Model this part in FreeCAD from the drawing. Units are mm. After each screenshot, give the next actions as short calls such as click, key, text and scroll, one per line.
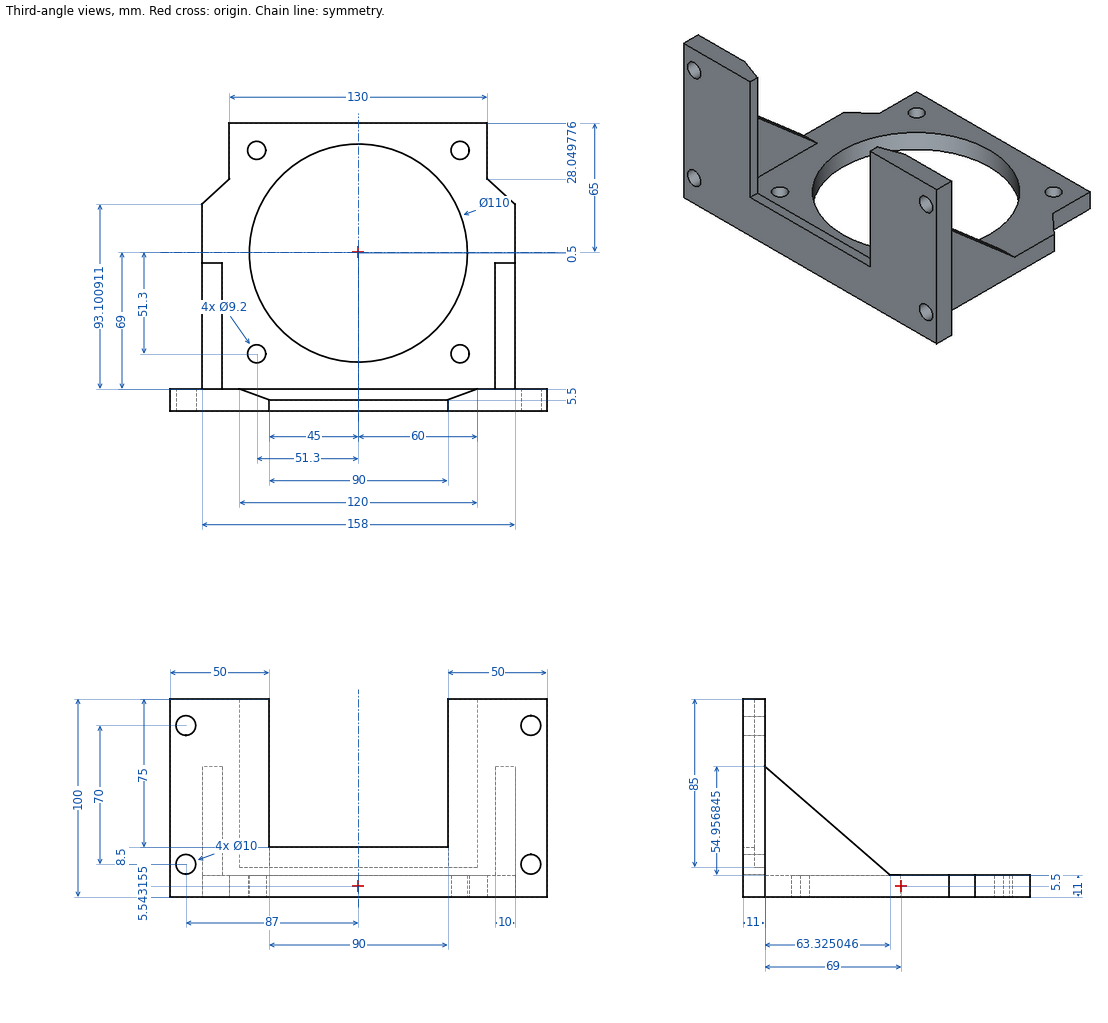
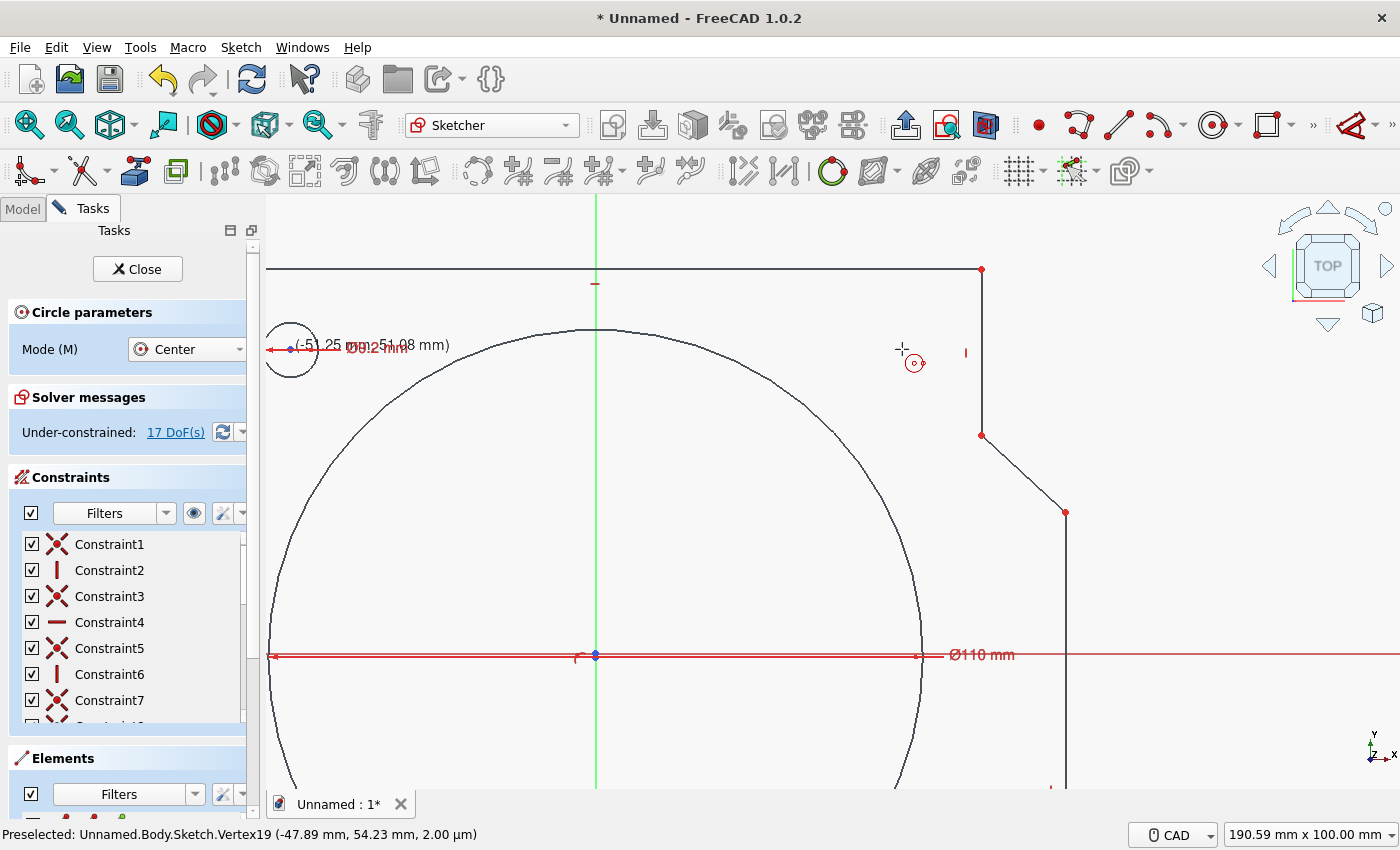
click(901, 349)
move(920, 329)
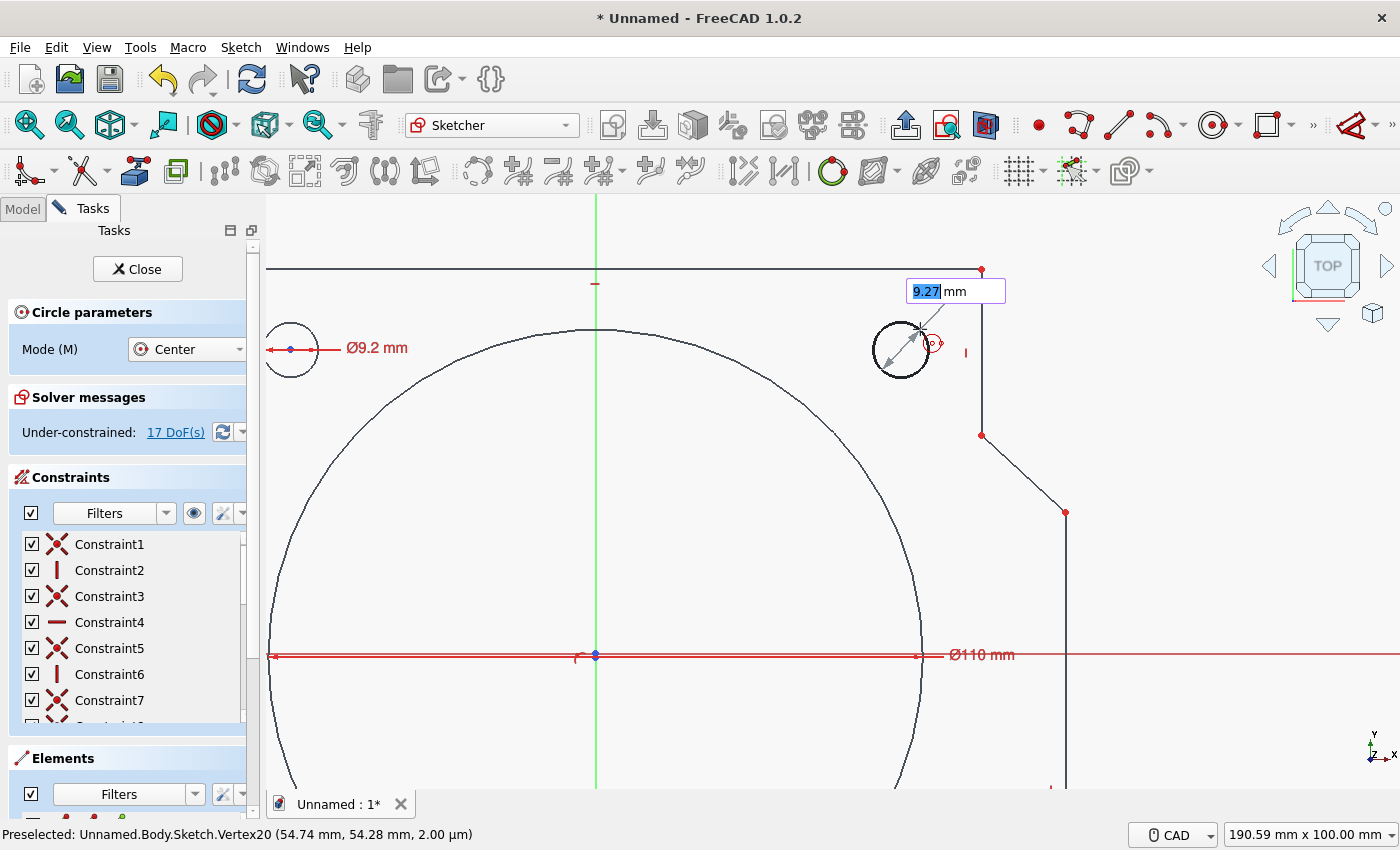
text(9.2)
key(Return)
key(Escape)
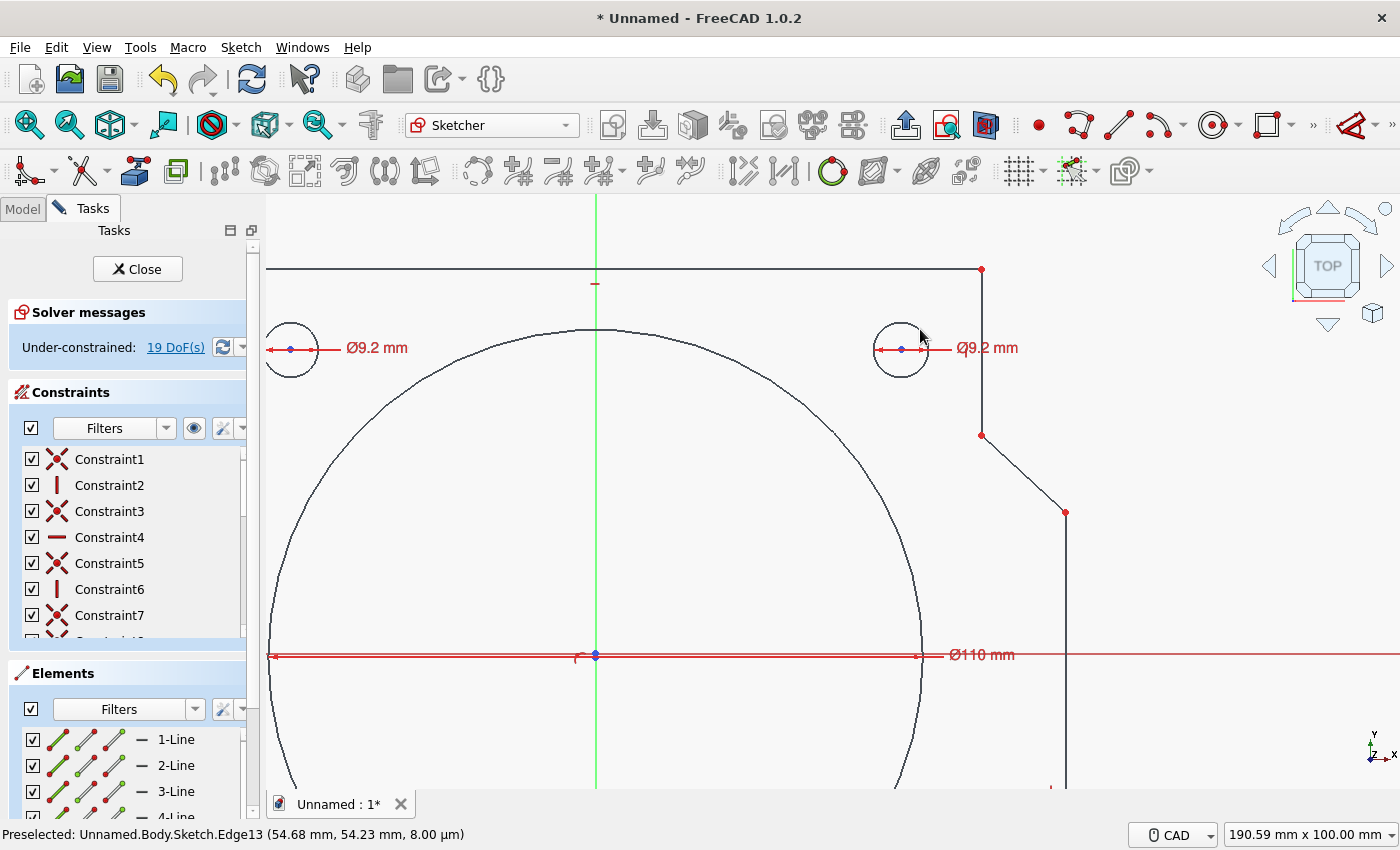
scroll(902, 349, down, 4)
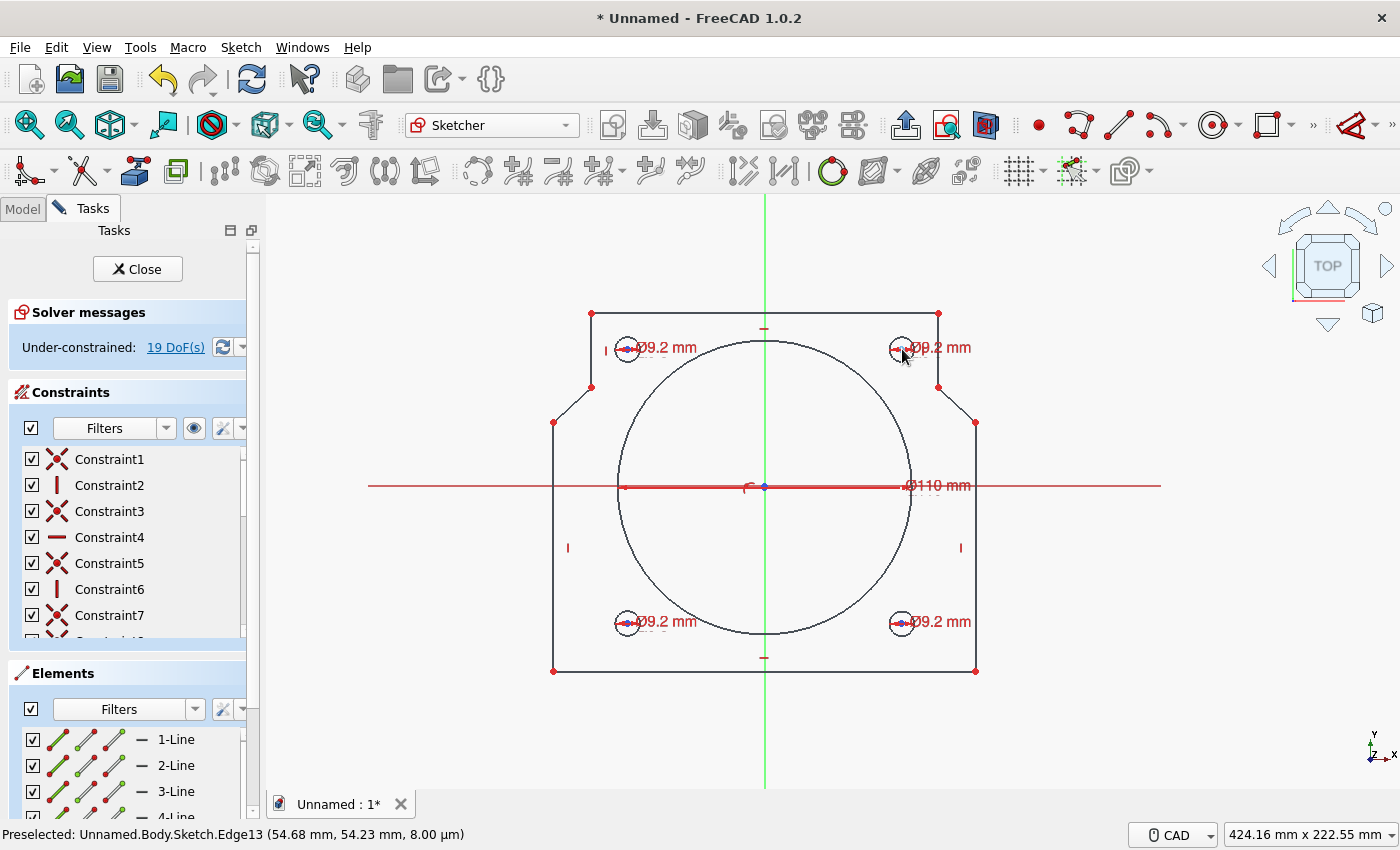
click(628, 624)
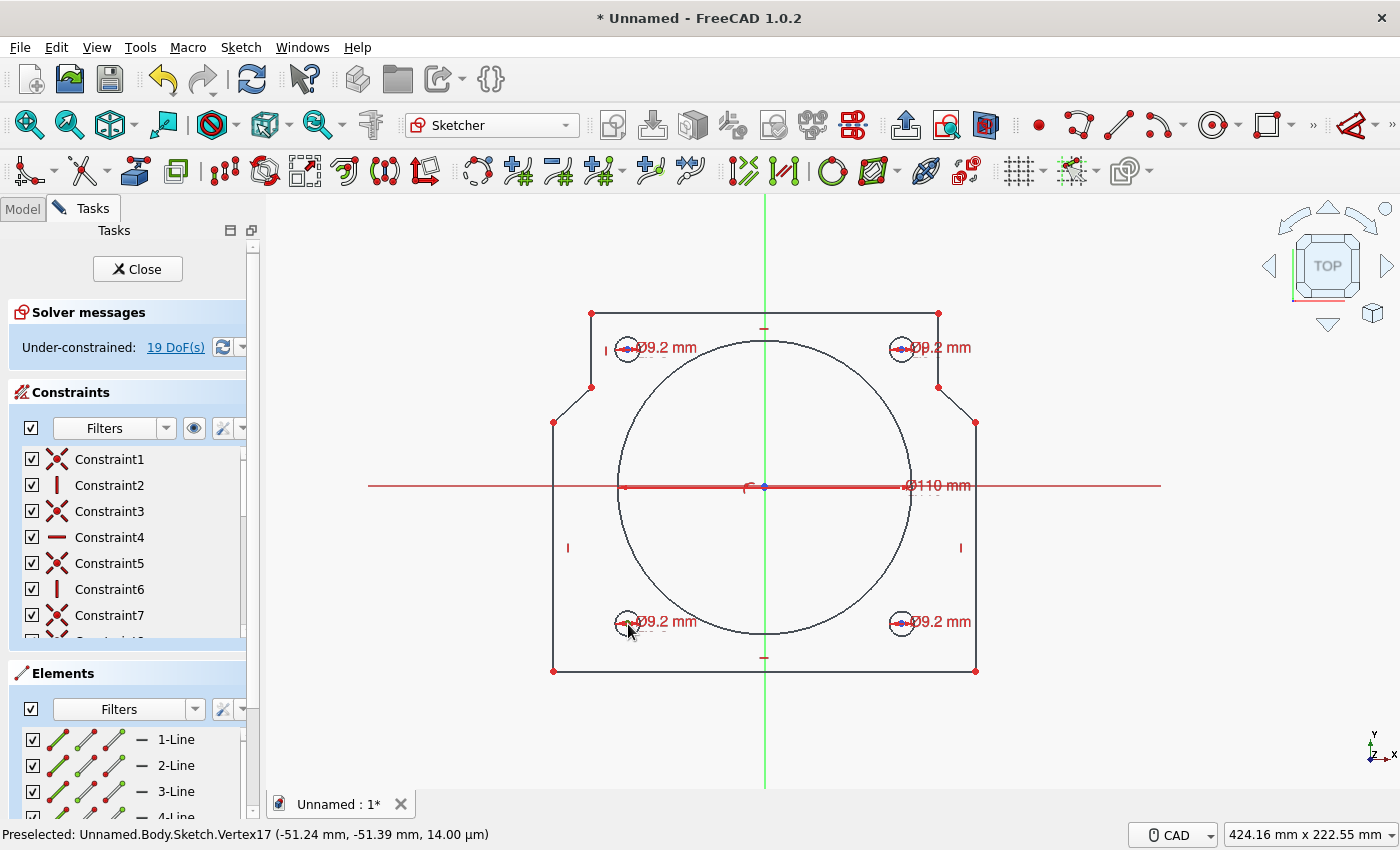
click(902, 624)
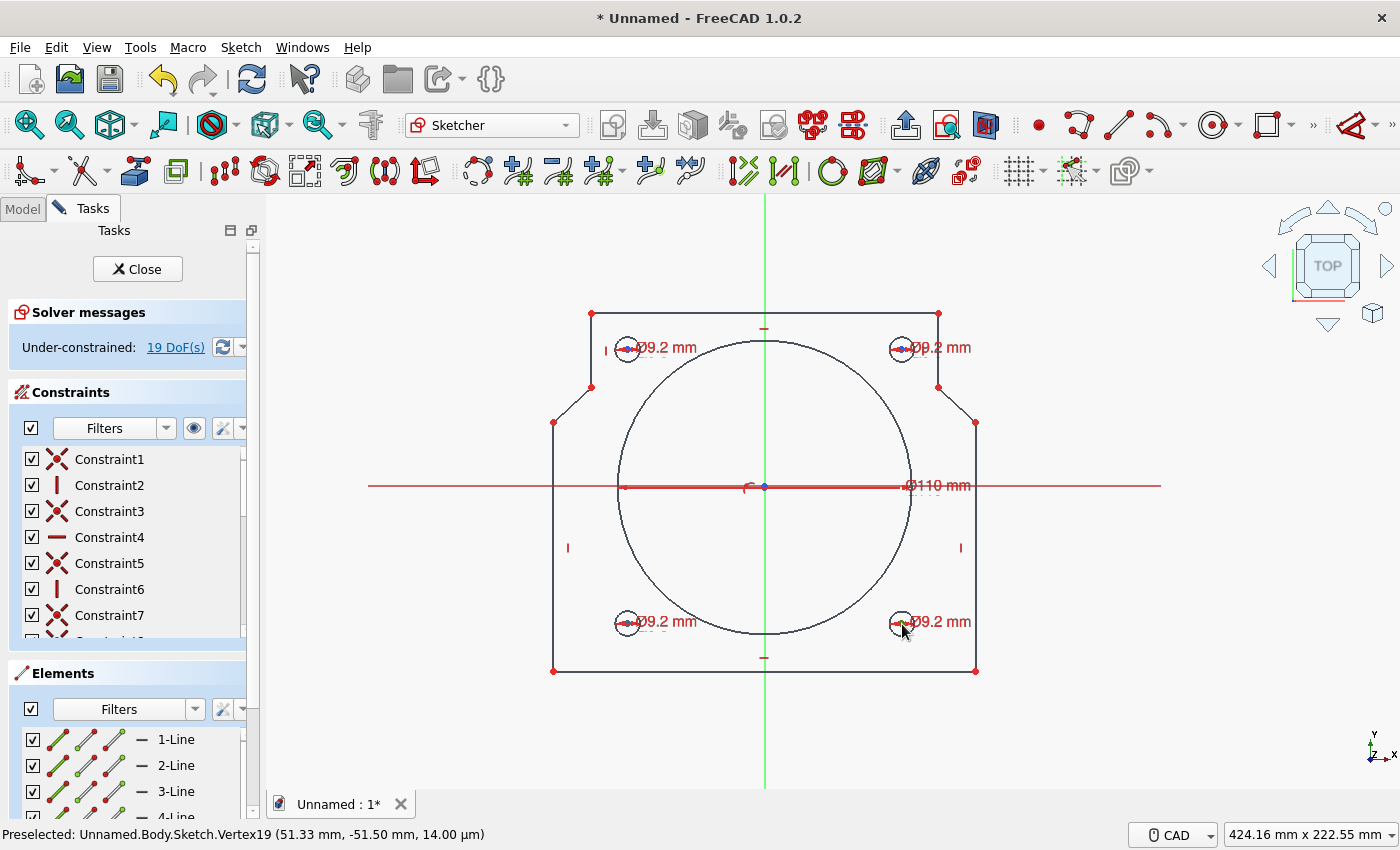
click(765, 722)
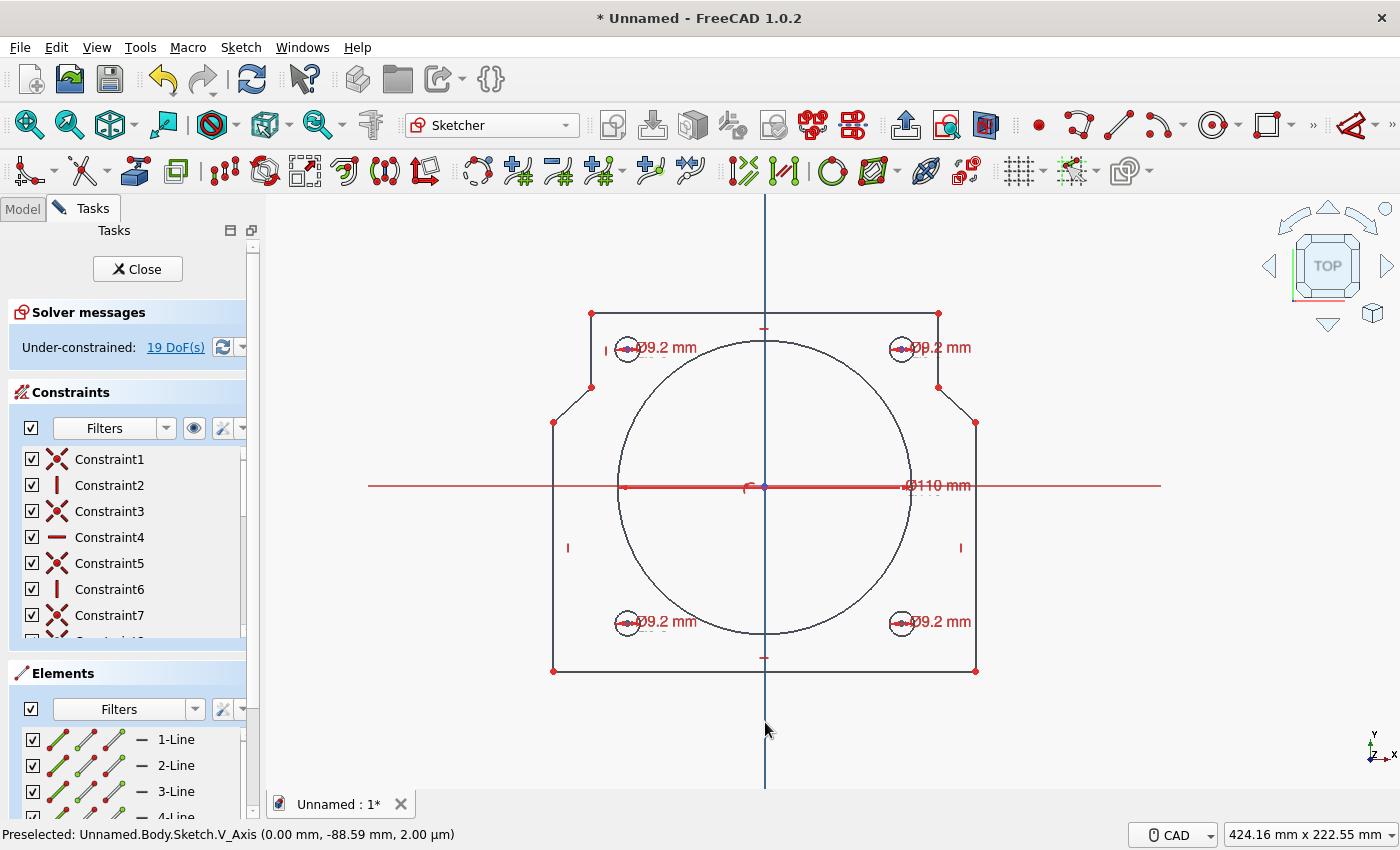
key(s)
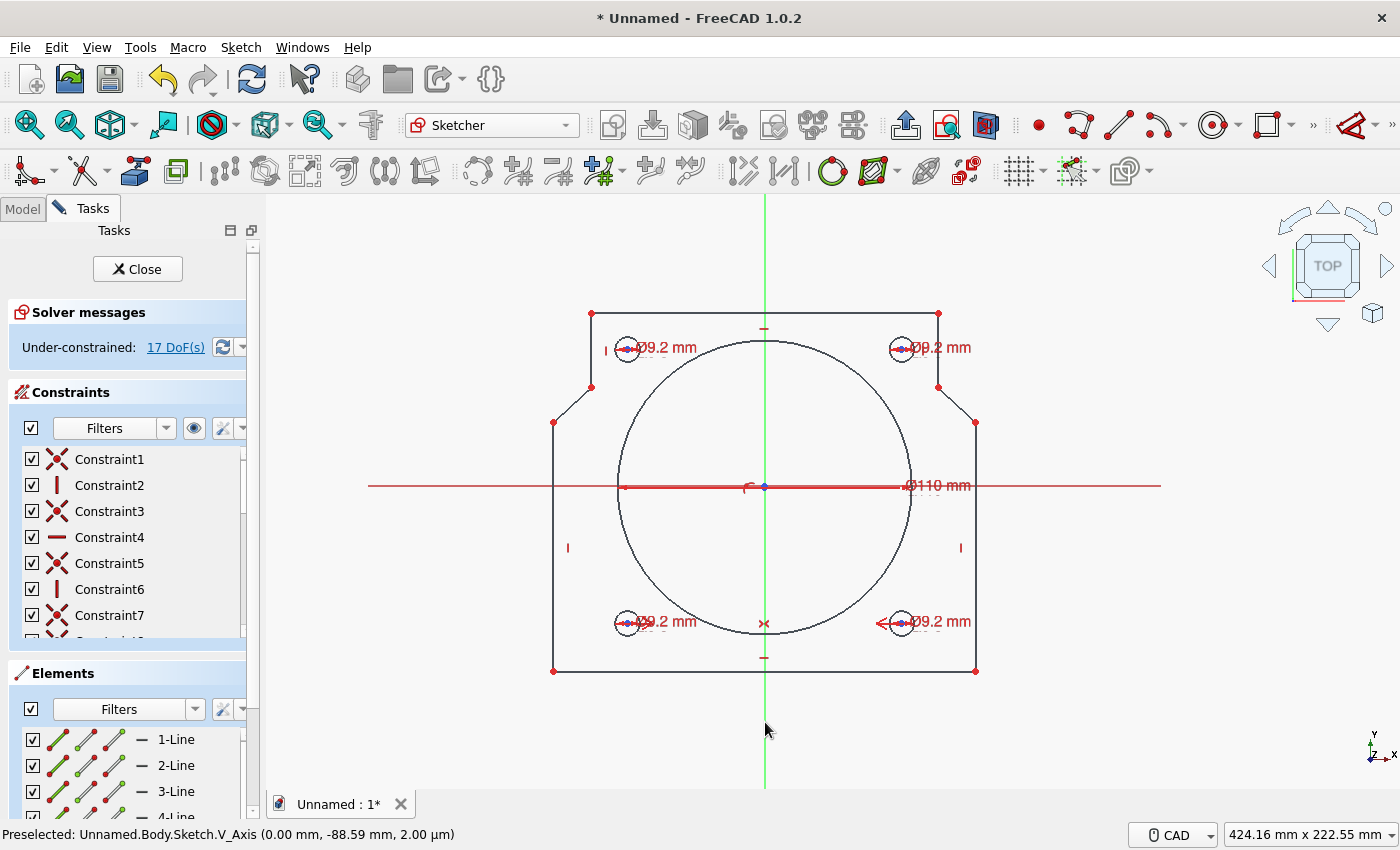
click(627, 624)